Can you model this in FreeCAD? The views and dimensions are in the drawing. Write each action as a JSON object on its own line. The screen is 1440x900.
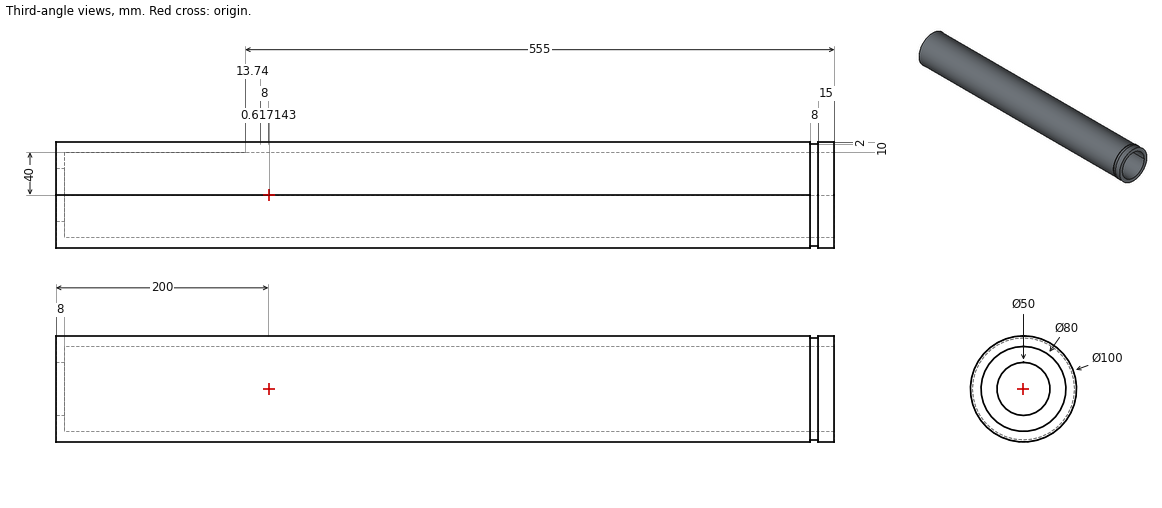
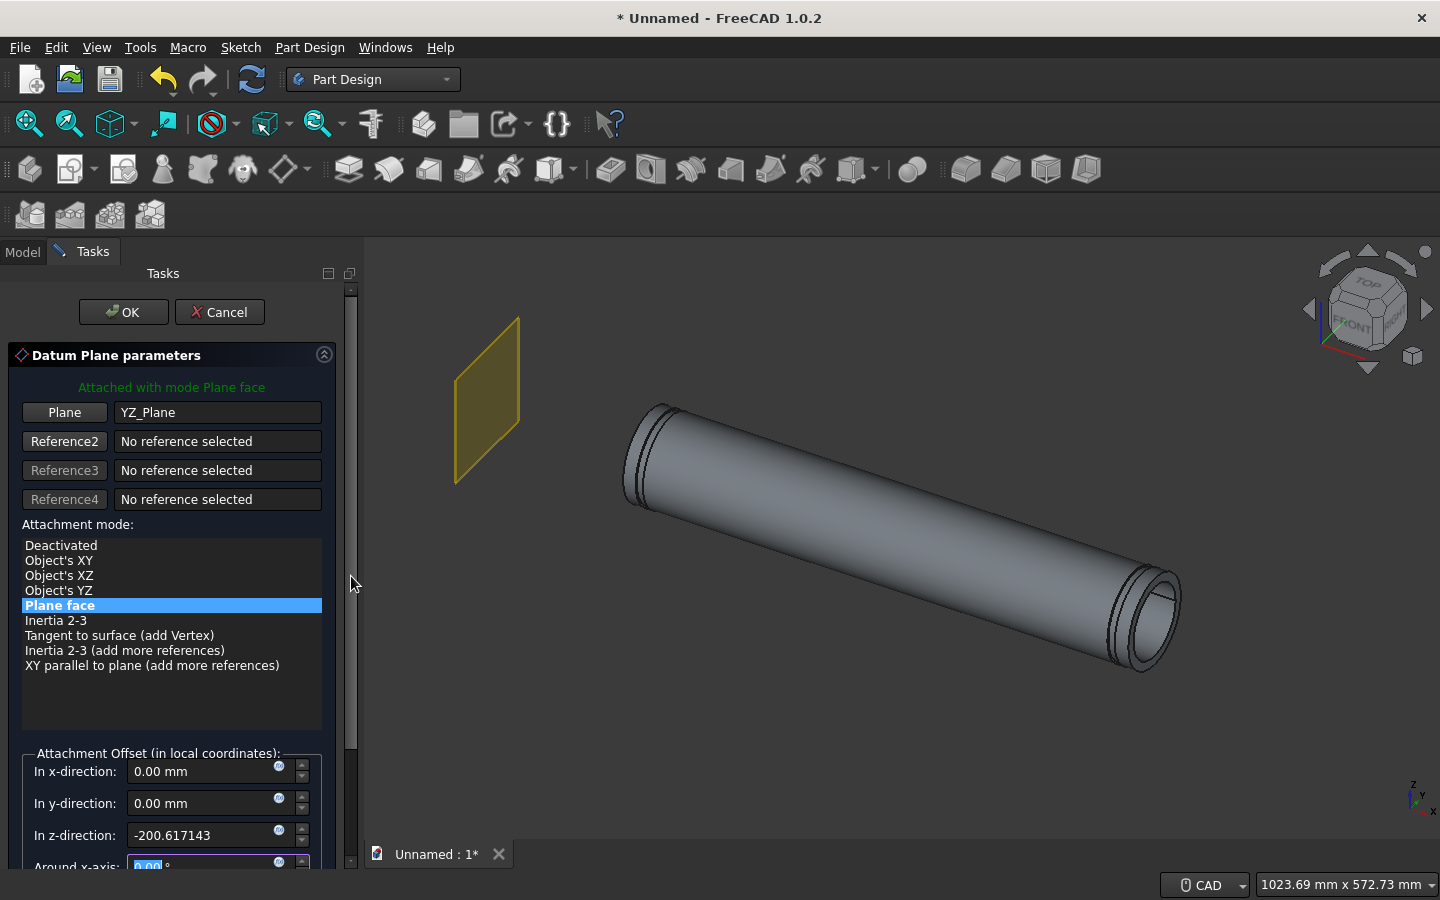
{"action": "left_click", "coordinate": [124, 312]}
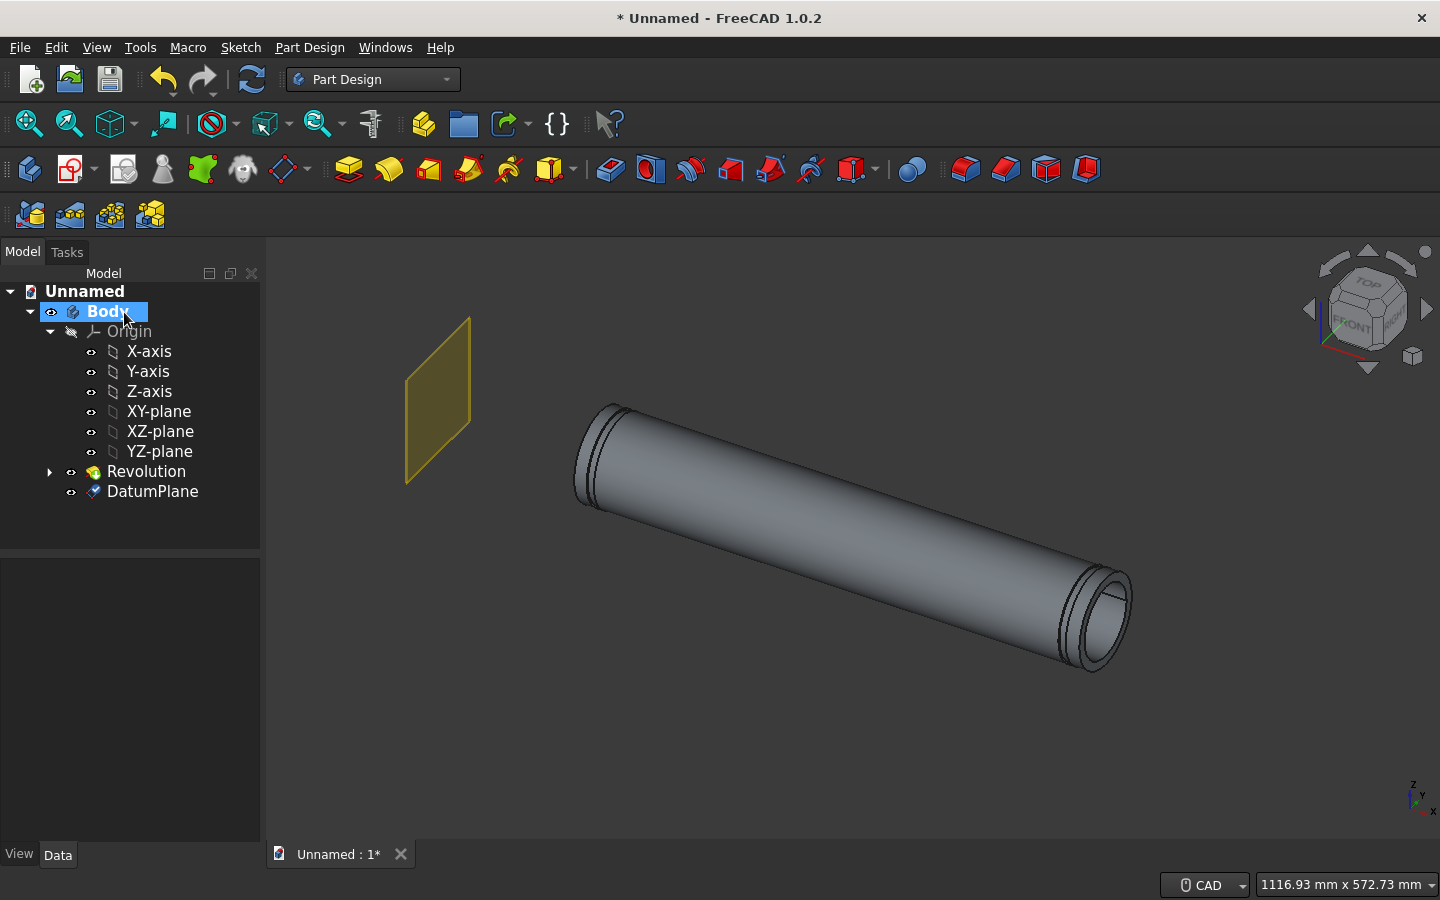
{"action": "left_click", "coordinate": [116, 492]}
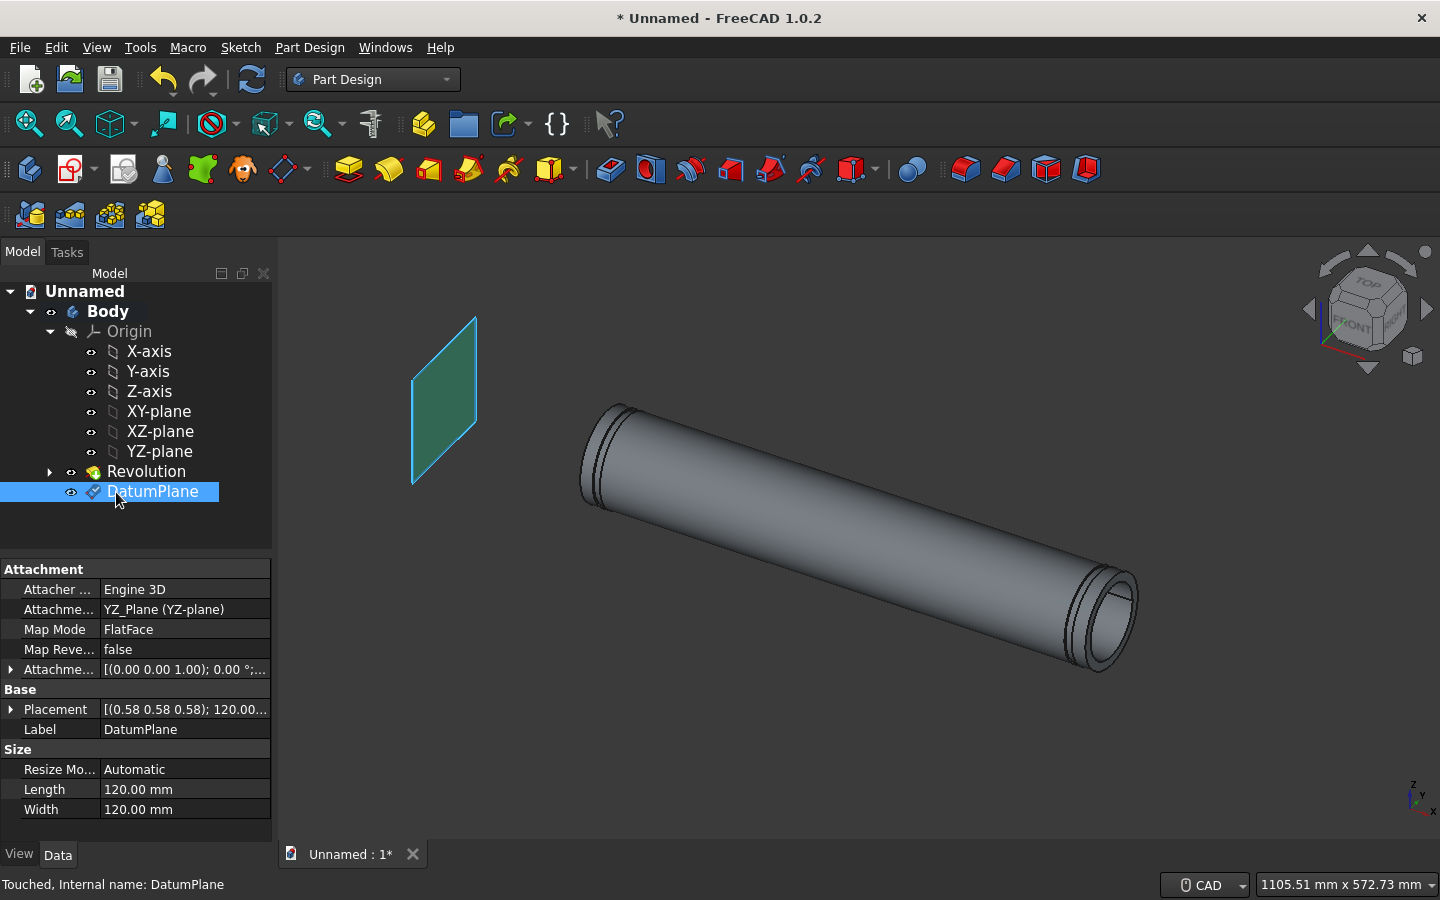
{"action": "left_click", "coordinate": [70, 170]}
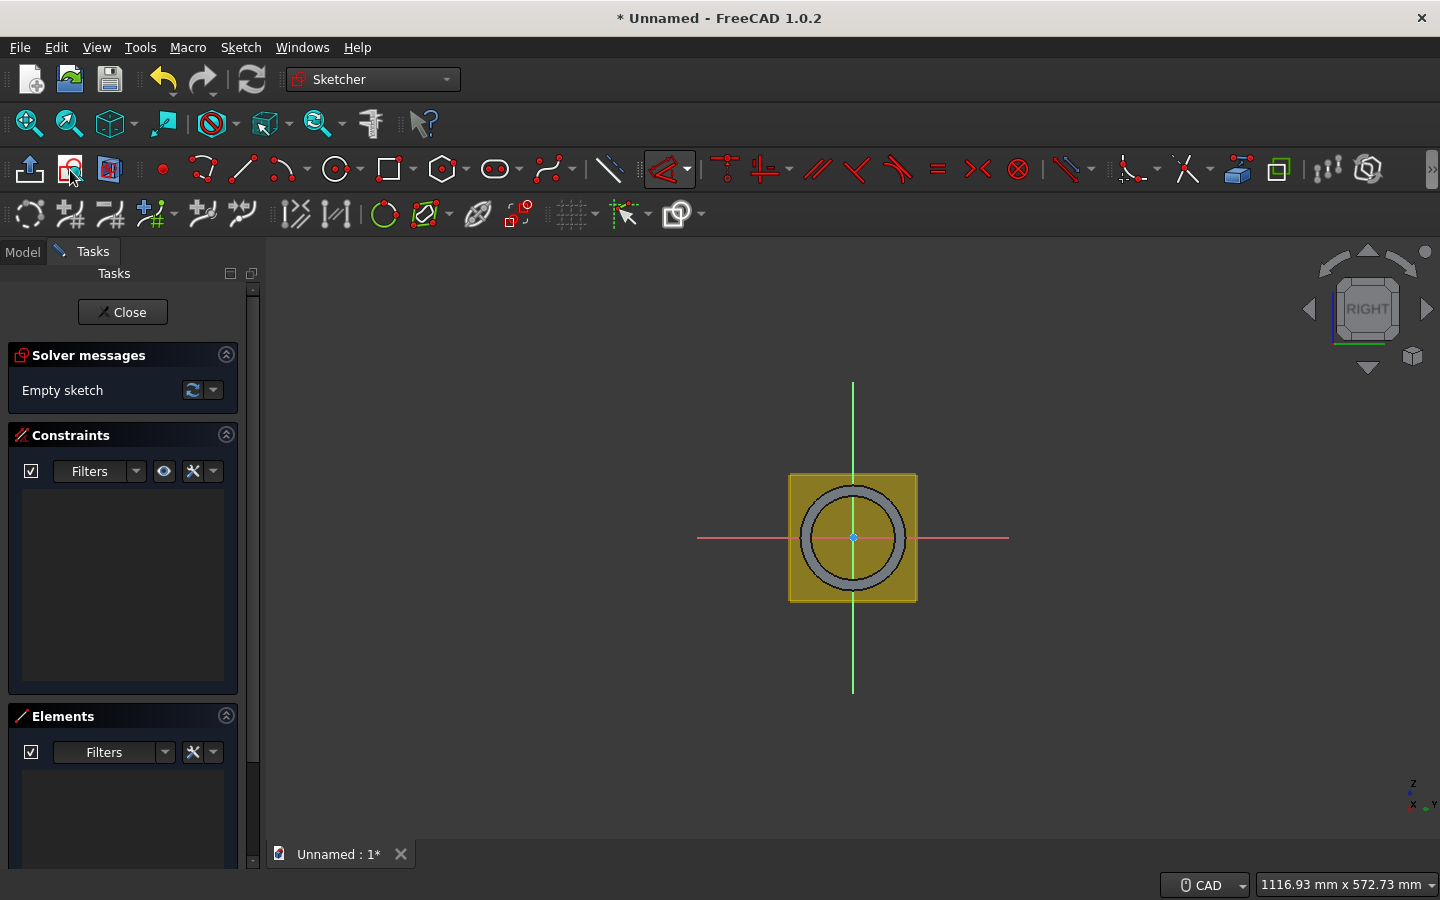
{"action": "key", "text": "q s"}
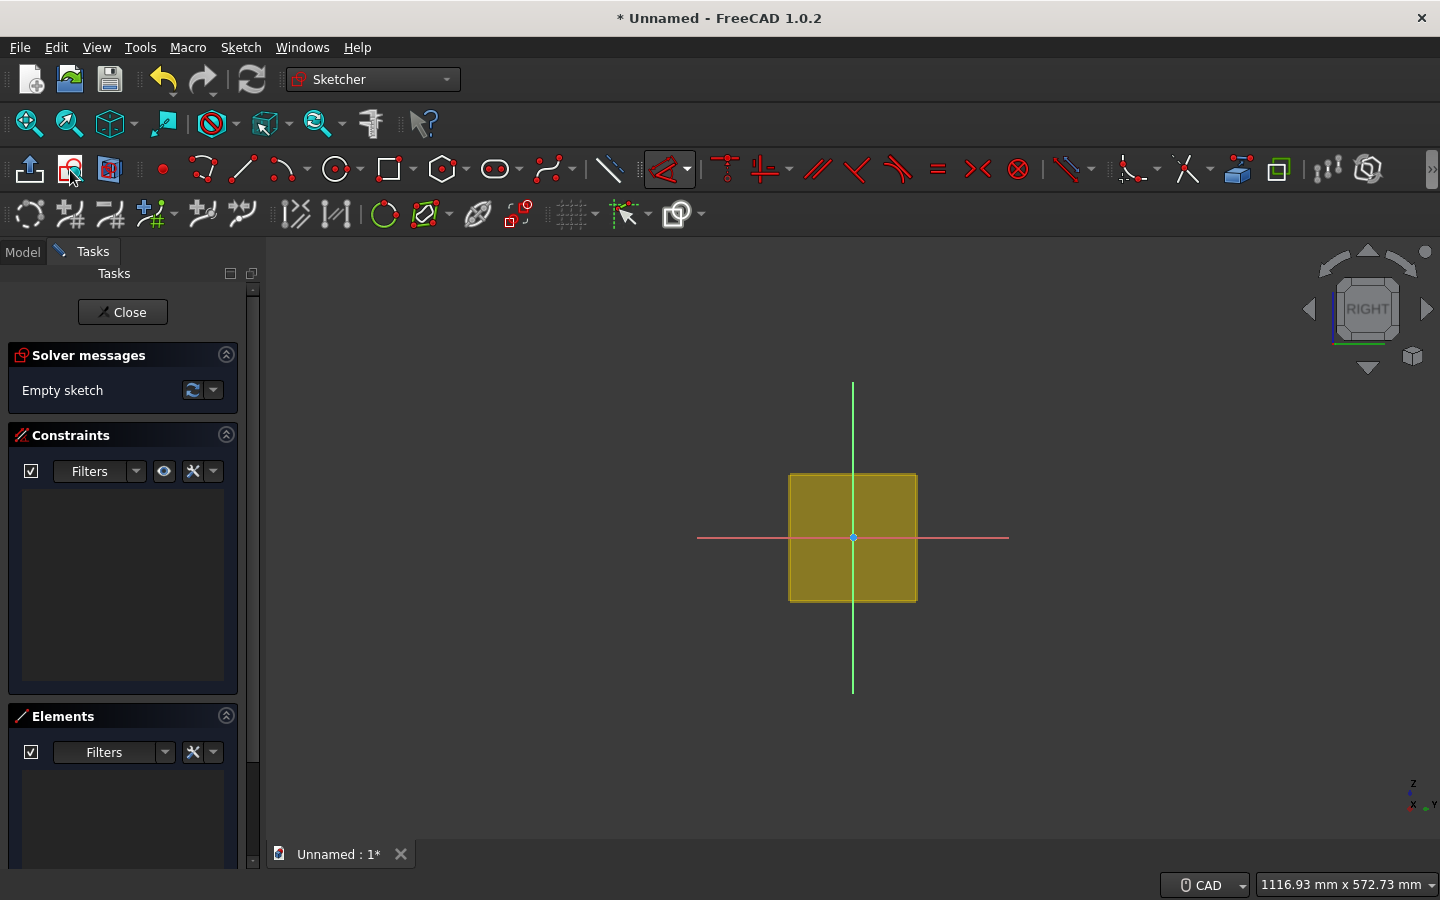
{"action": "scroll", "coordinate": [883, 538], "scroll_direction": "up", "scroll_amount": 6}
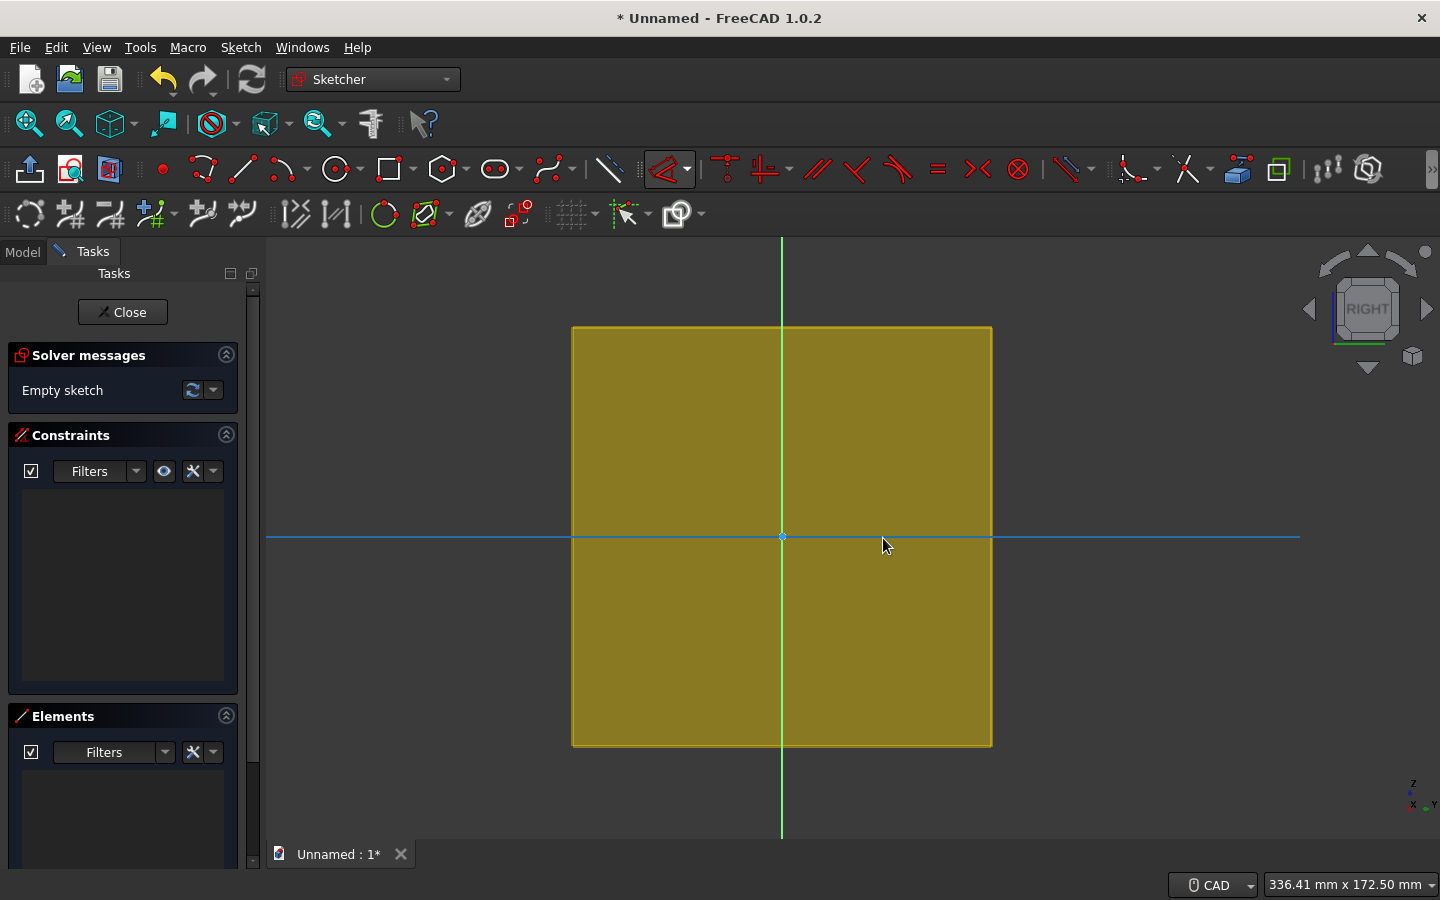
{"action": "key", "text": "g c"}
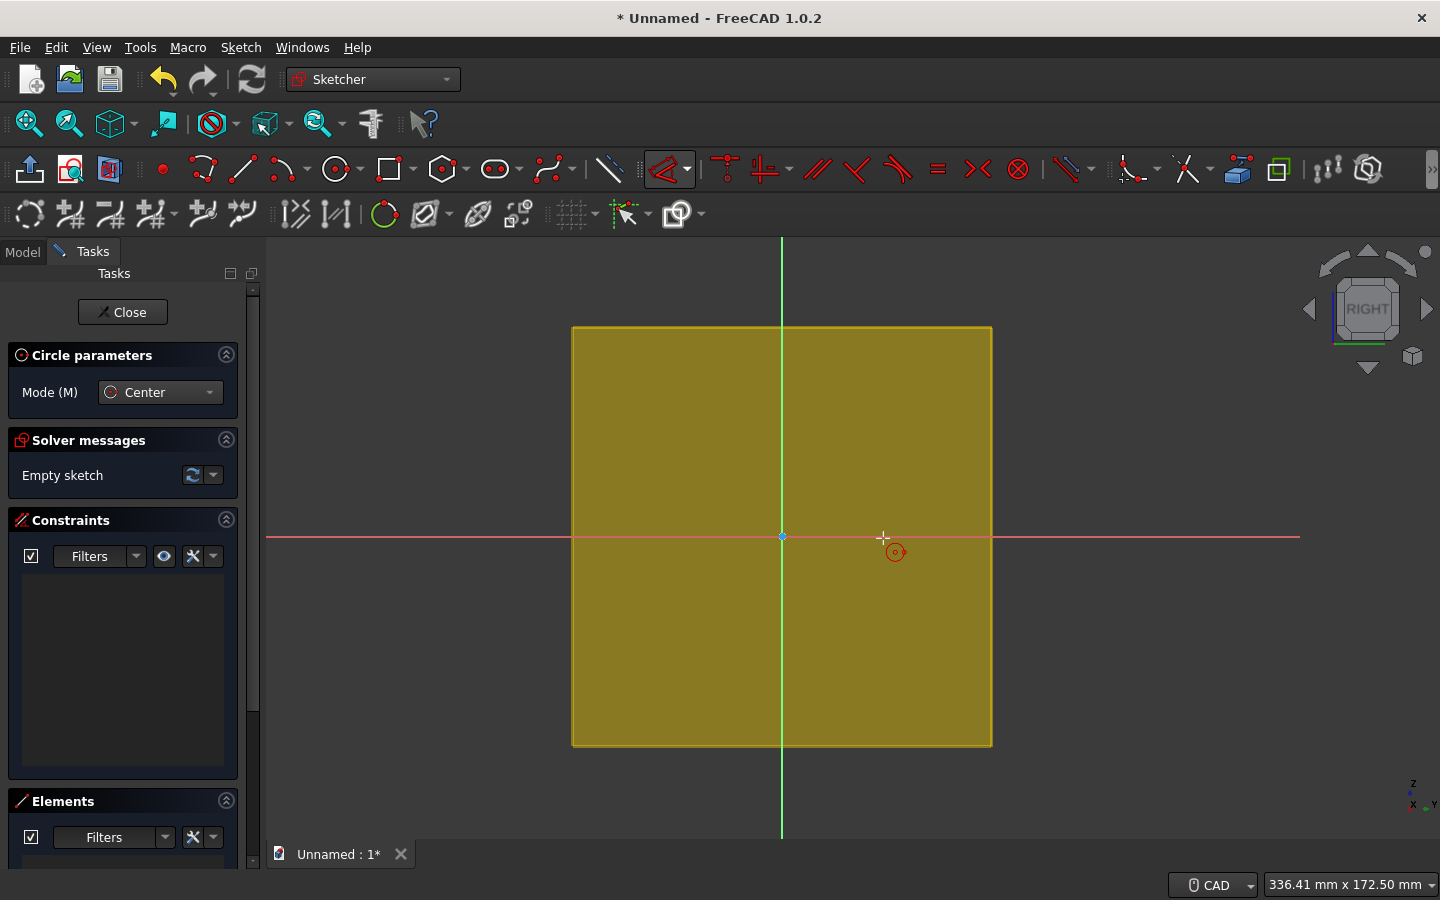
{"action": "left_click", "coordinate": [782, 537]}
{"action": "mouse_move", "coordinate": [906, 413]}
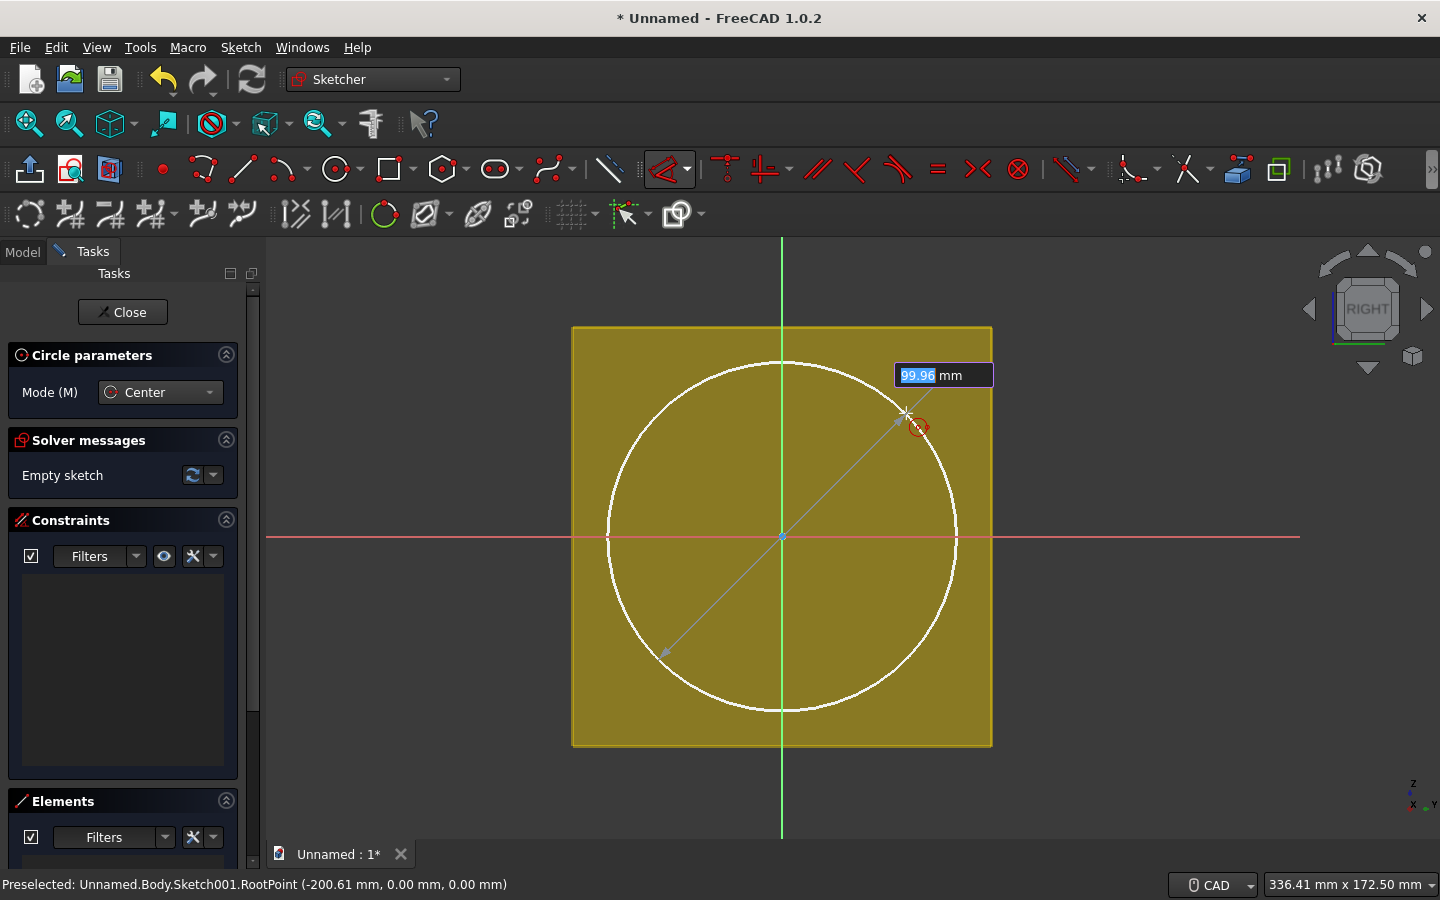
{"action": "type", "text": "100"}
{"action": "key", "text": "Return"}